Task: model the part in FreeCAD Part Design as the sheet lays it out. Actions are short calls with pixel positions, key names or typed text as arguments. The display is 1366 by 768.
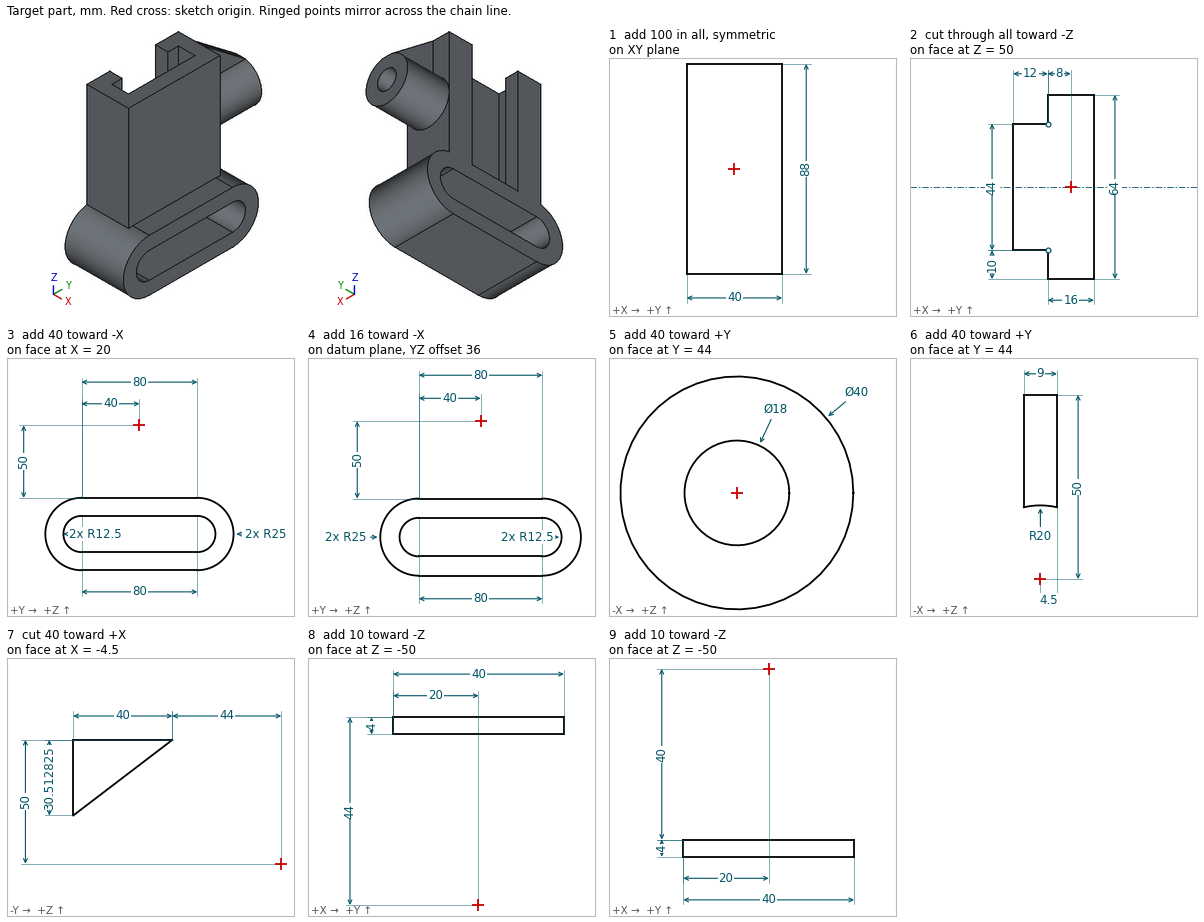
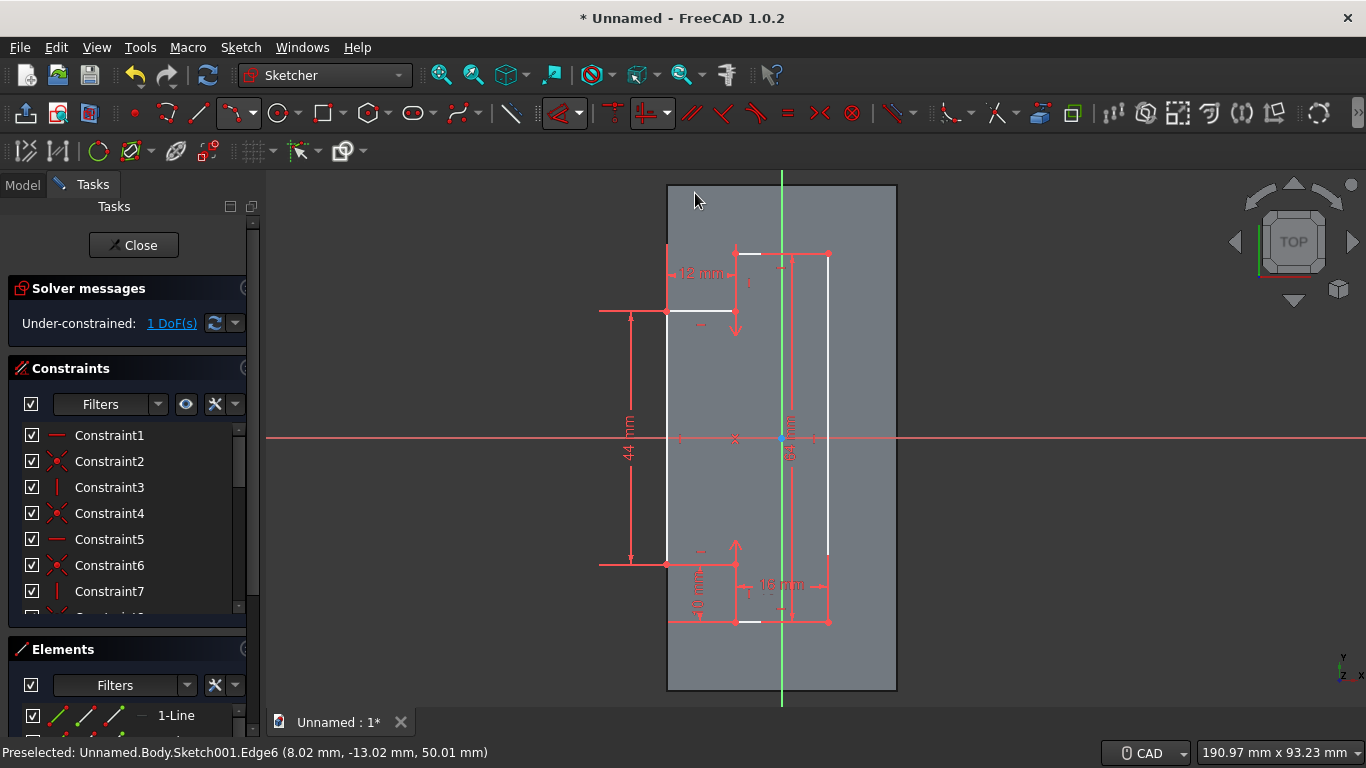
click(736, 311)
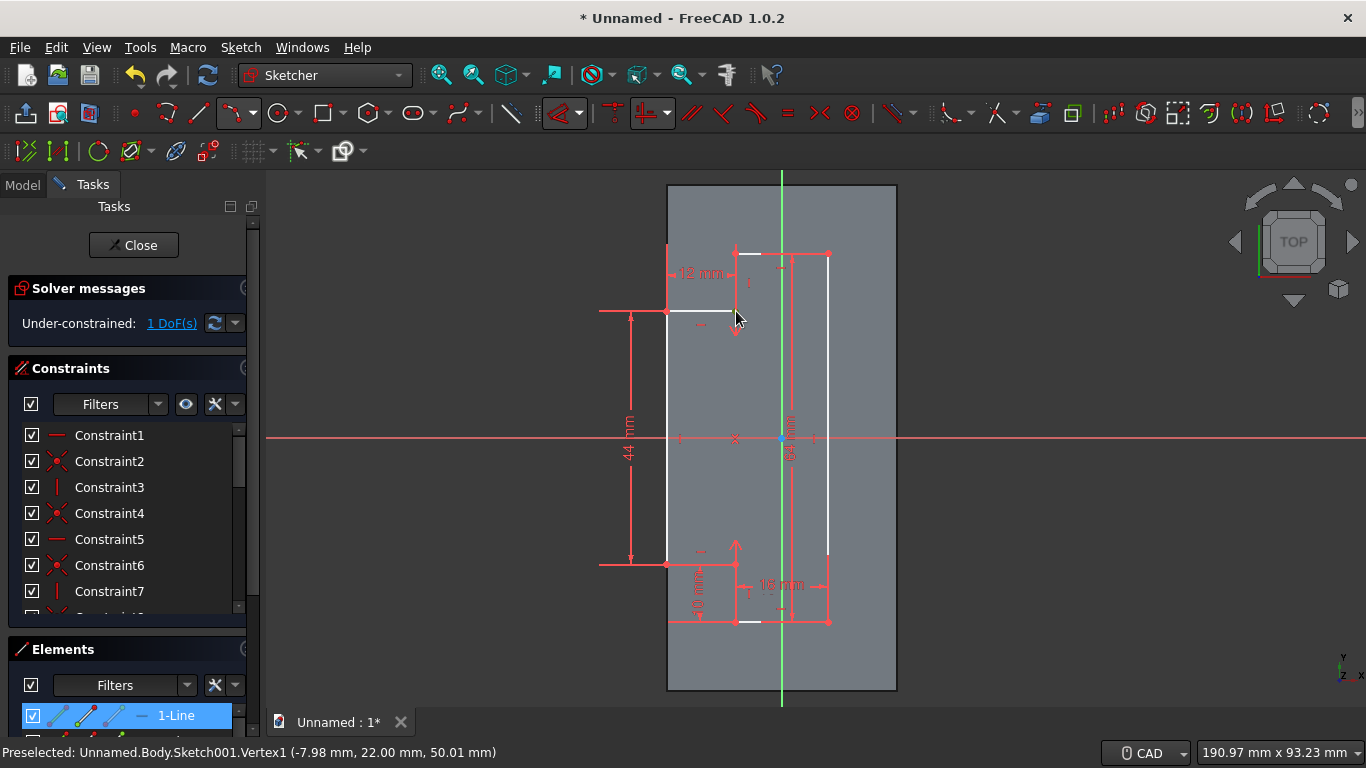
key(l)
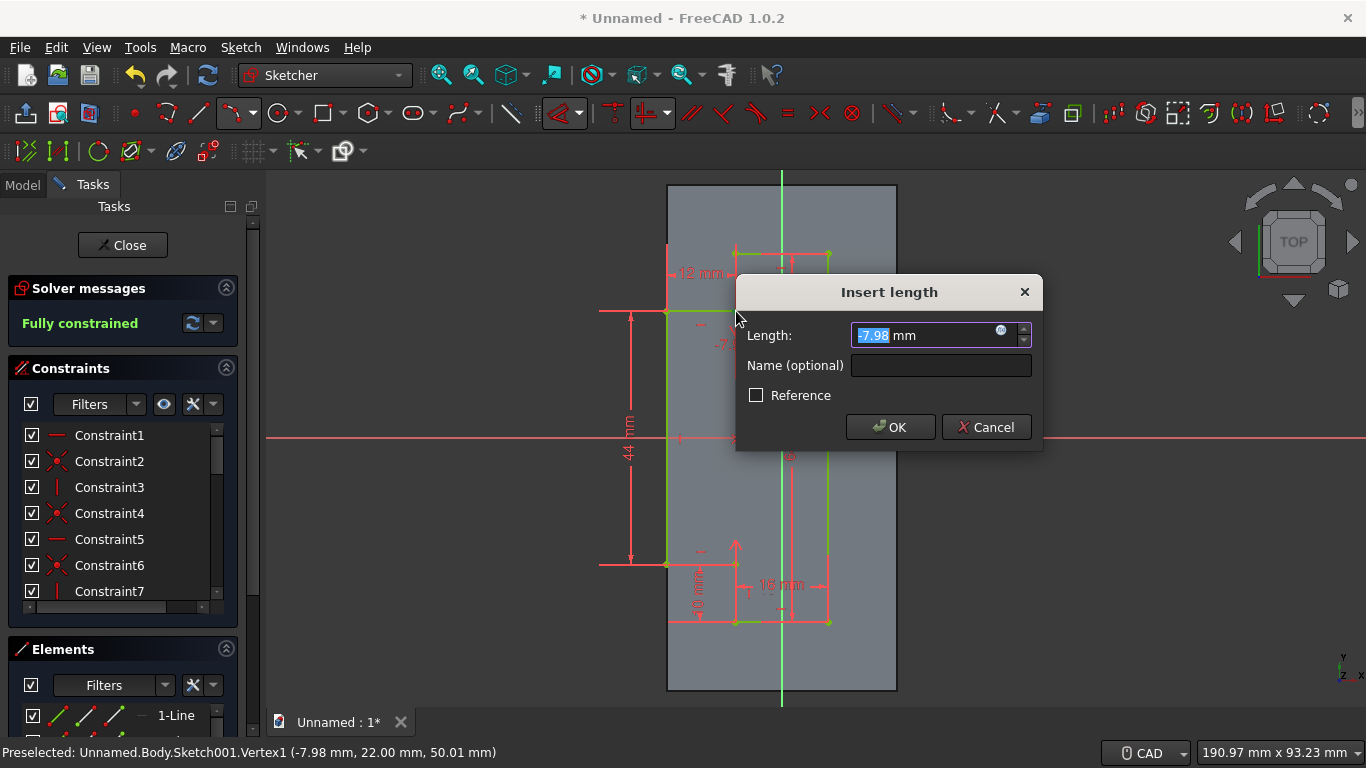
text(-8)
key(Return)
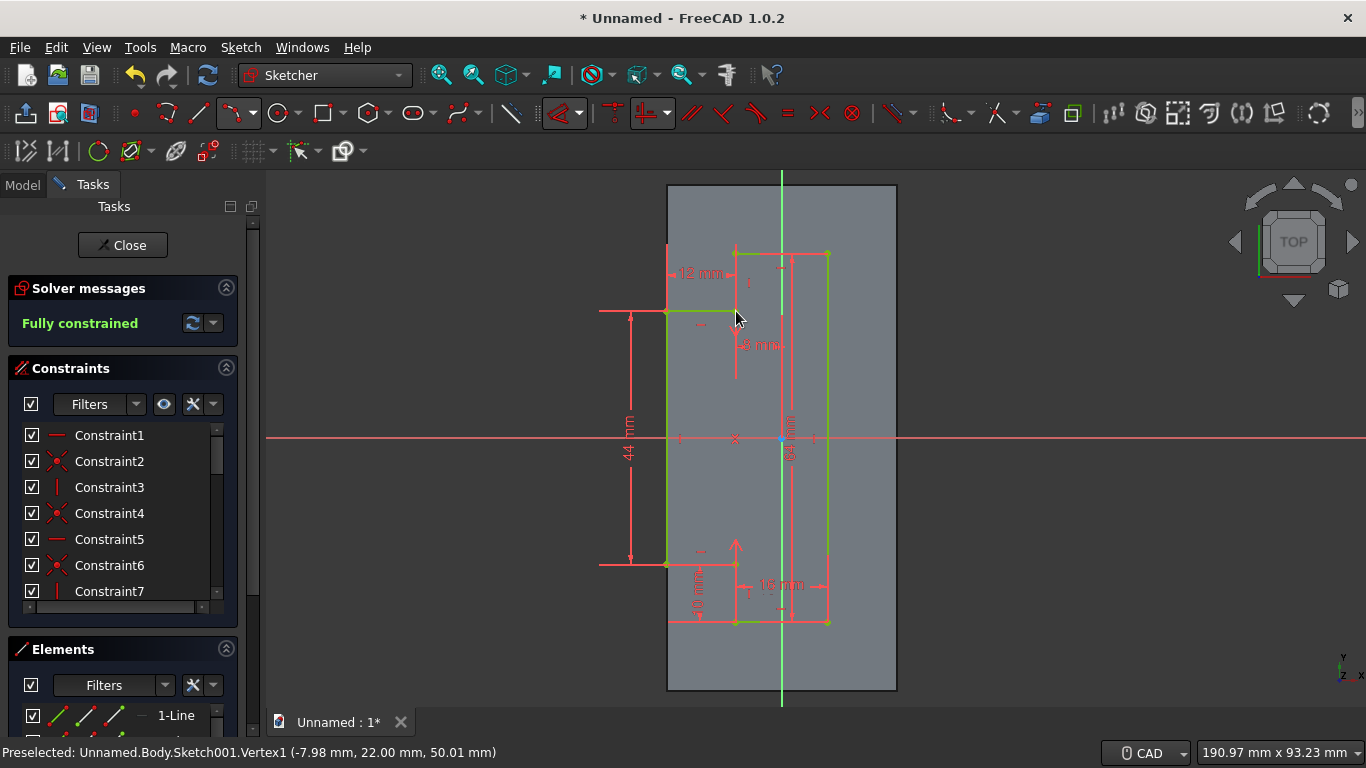
click(123, 245)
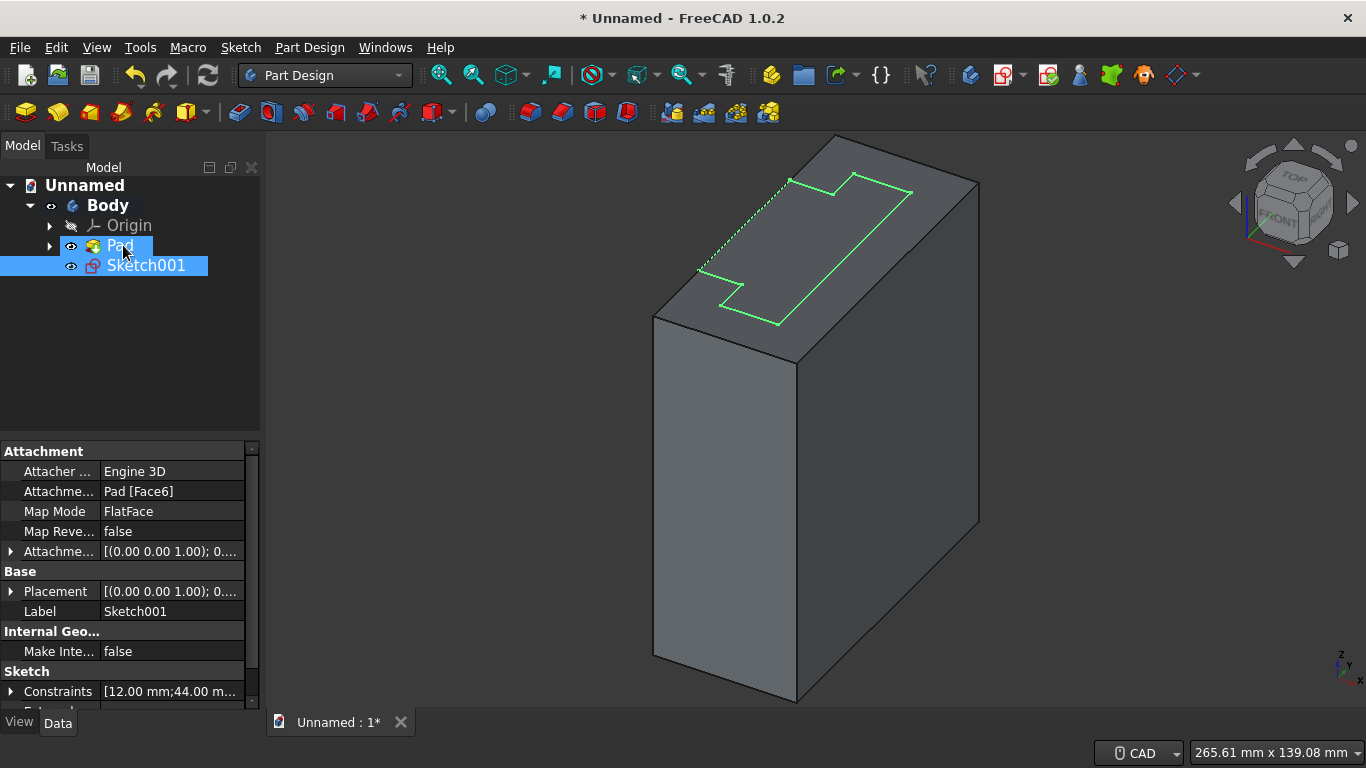
click(240, 112)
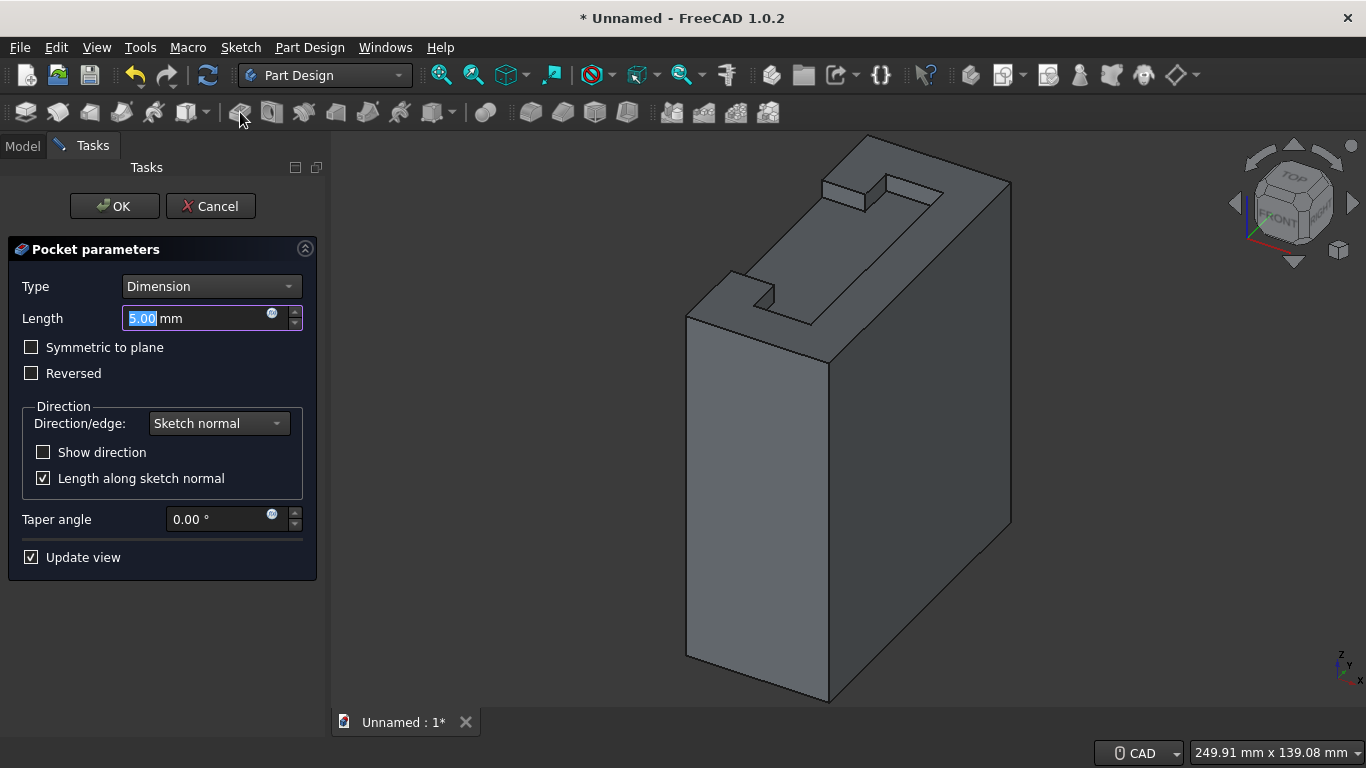
click(212, 286)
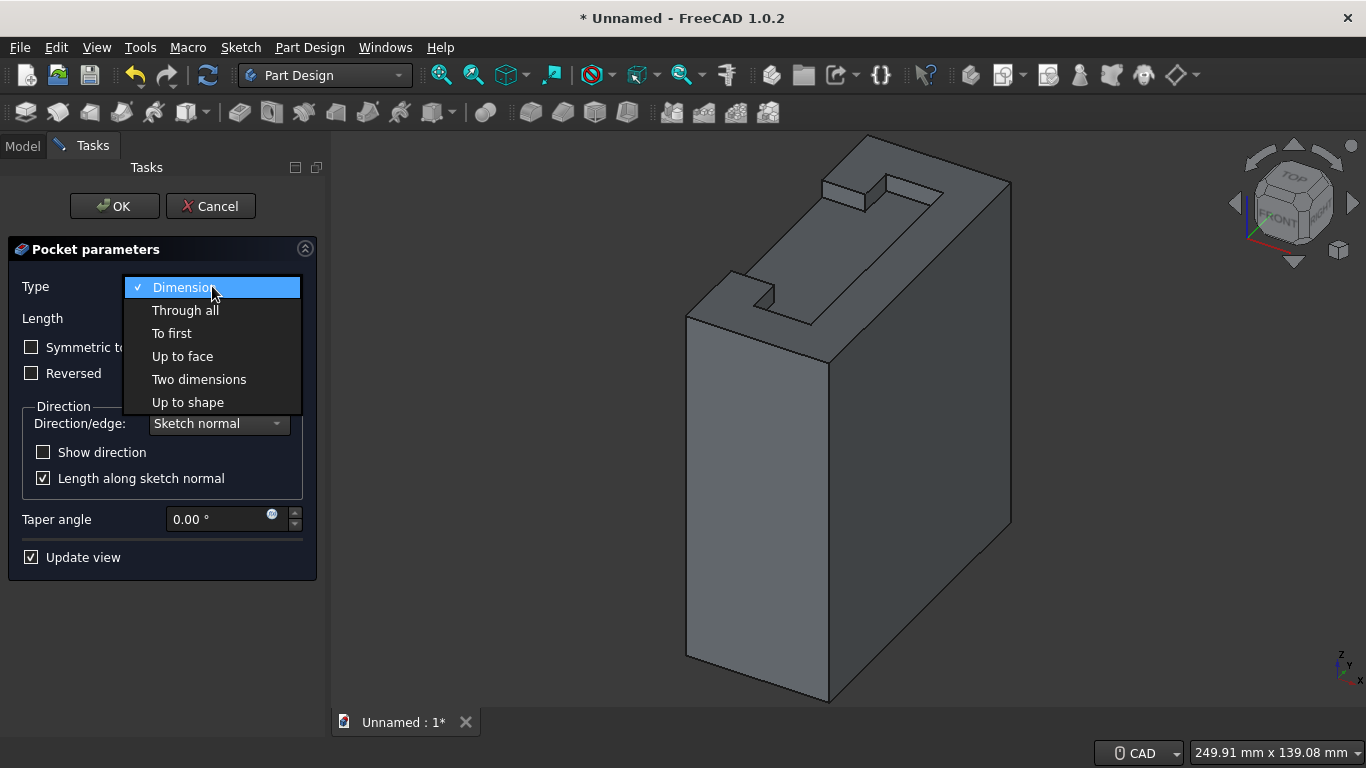
click(212, 310)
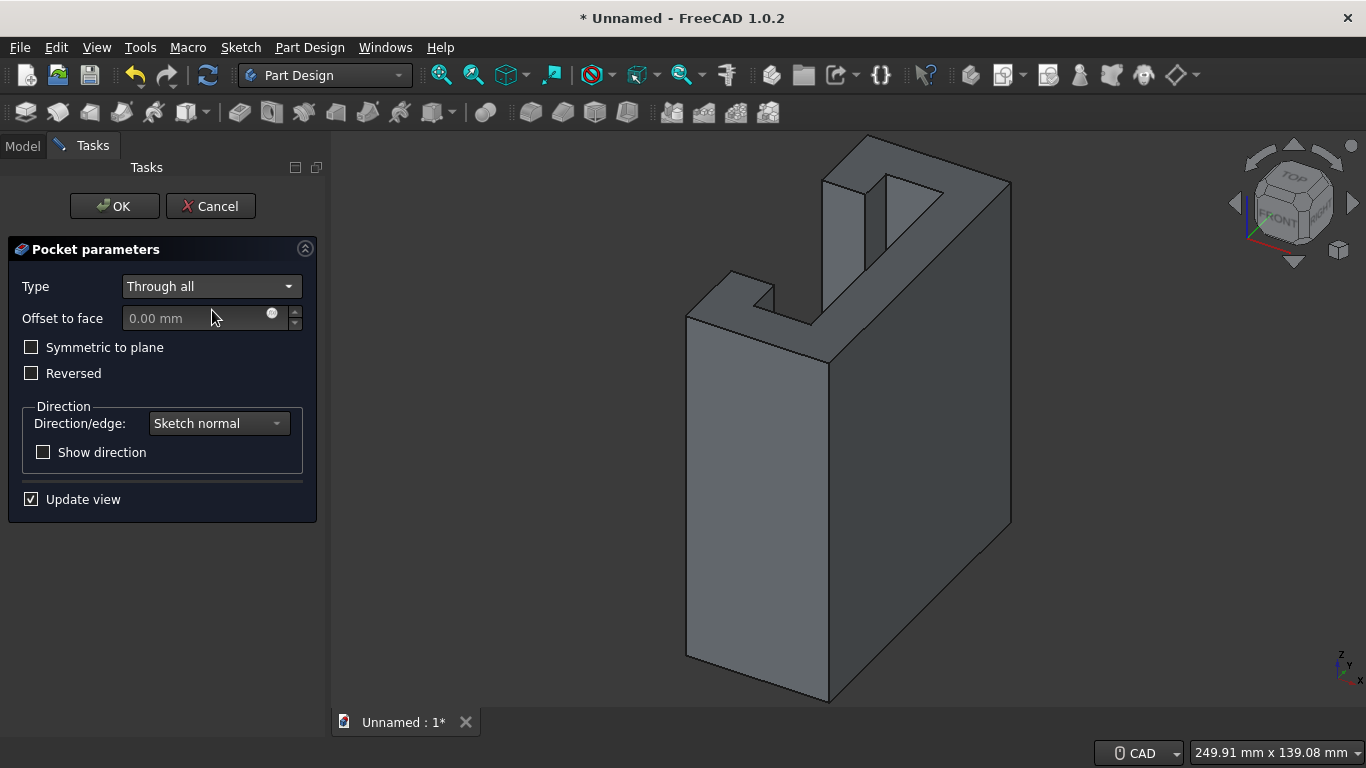
click(115, 206)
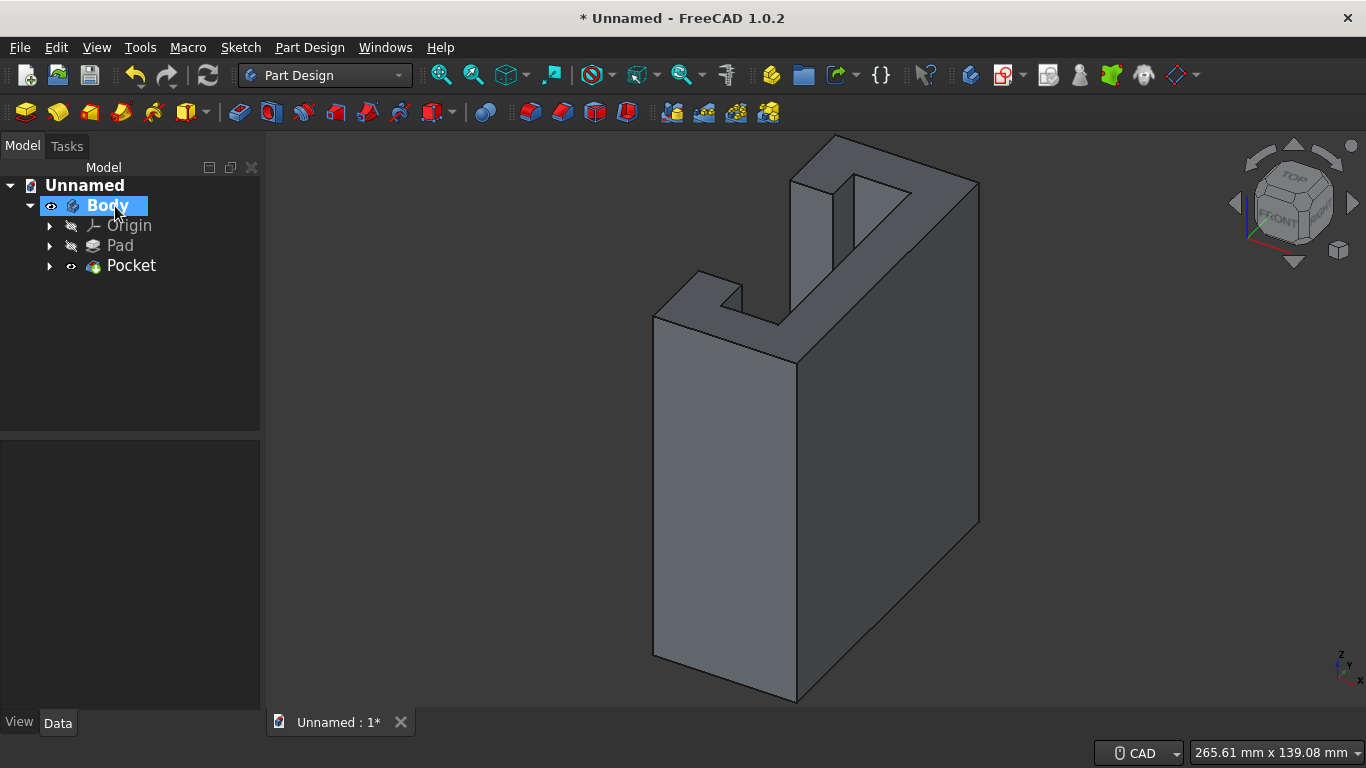
click(888, 442)